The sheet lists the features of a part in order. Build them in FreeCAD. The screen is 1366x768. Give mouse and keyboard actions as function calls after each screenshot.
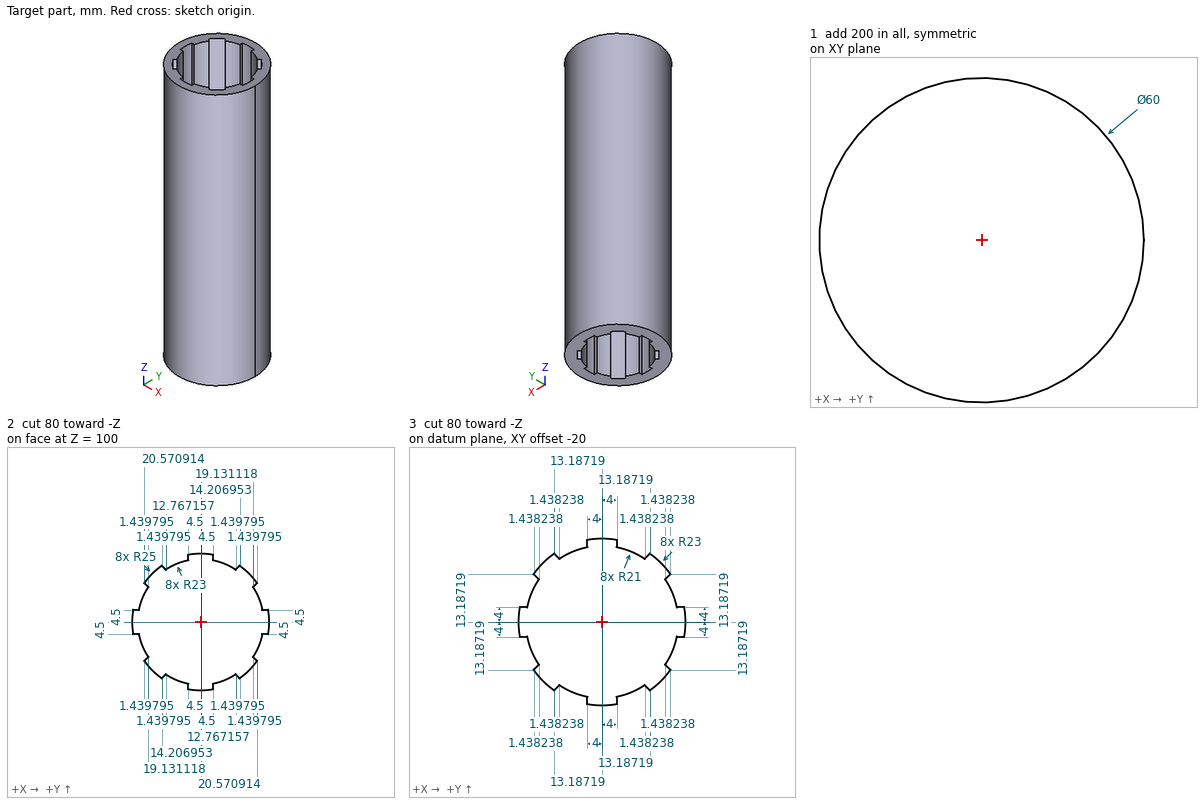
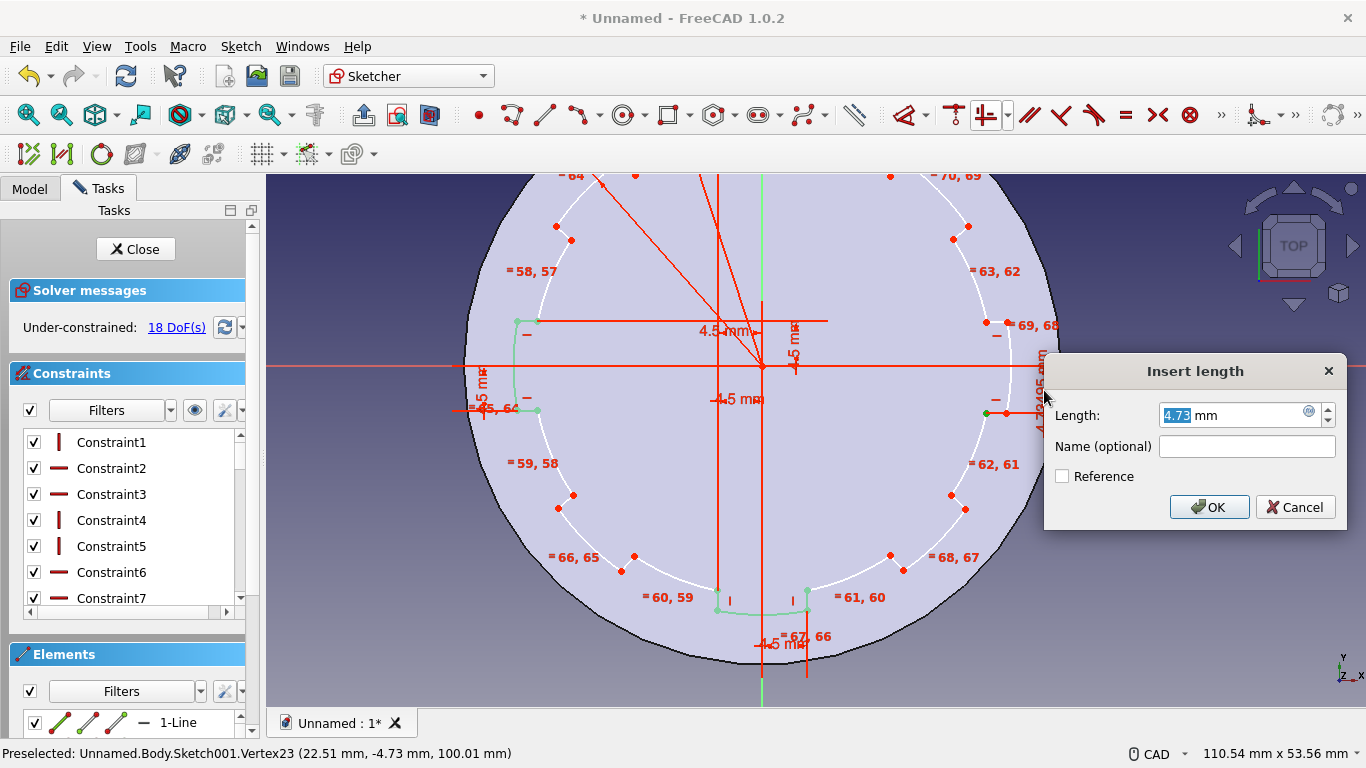
text(4.5)
key(Return)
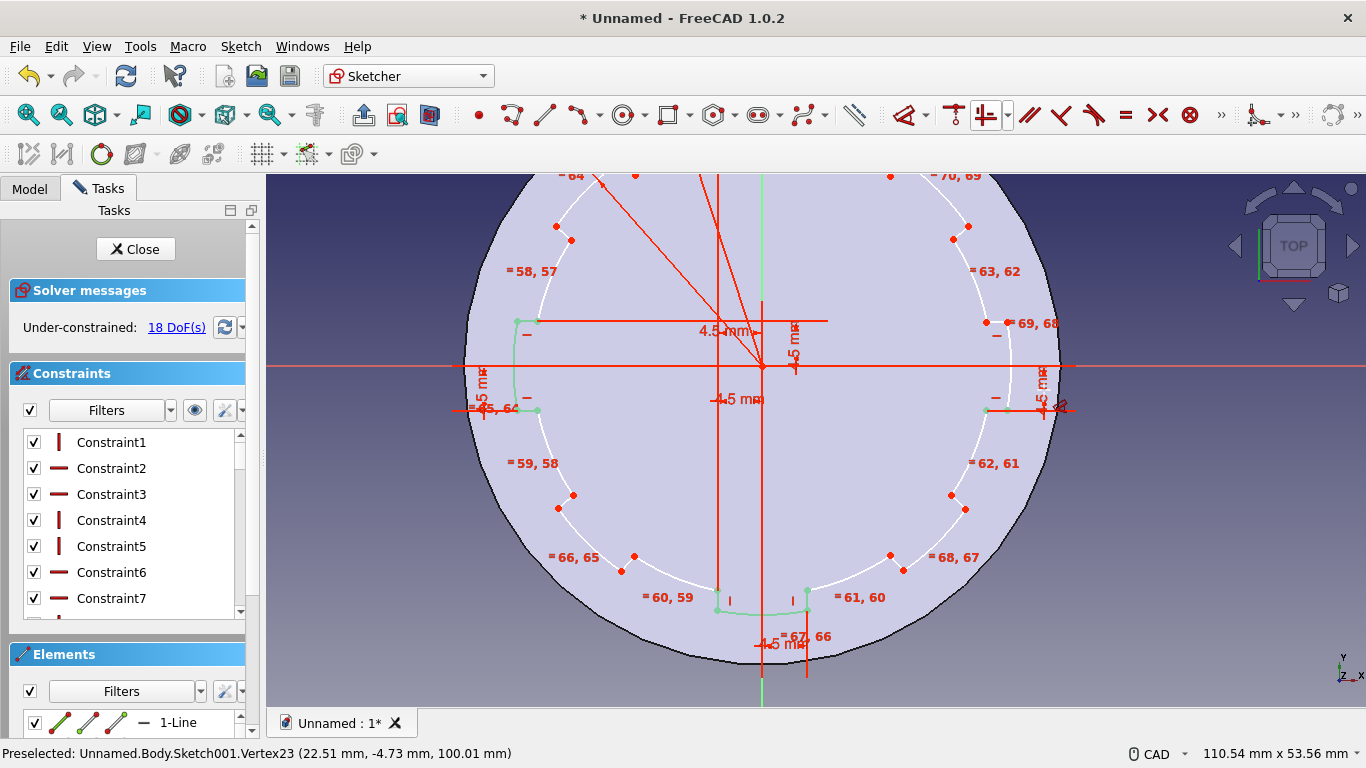
click(1007, 322)
click(1041, 344)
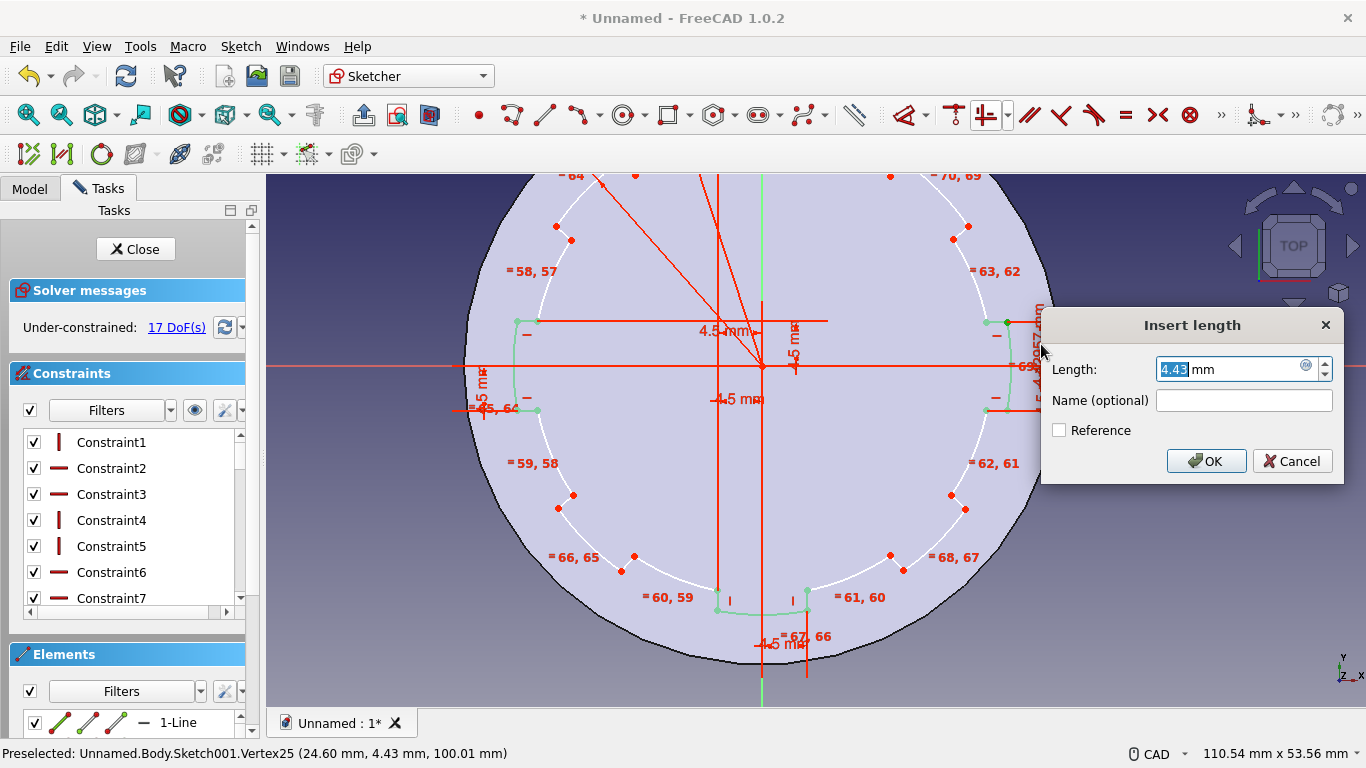
text(4.5)
key(Return)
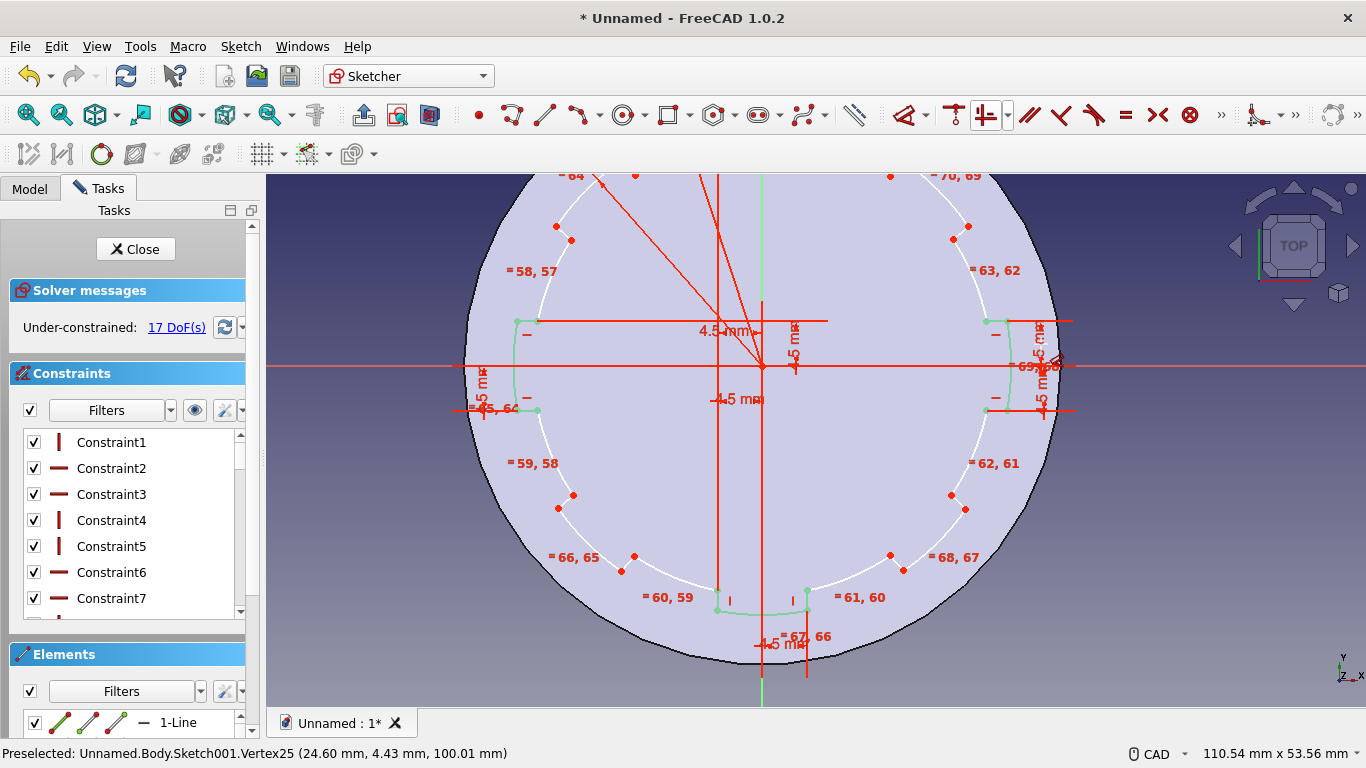
scroll(717, 592, down, 2)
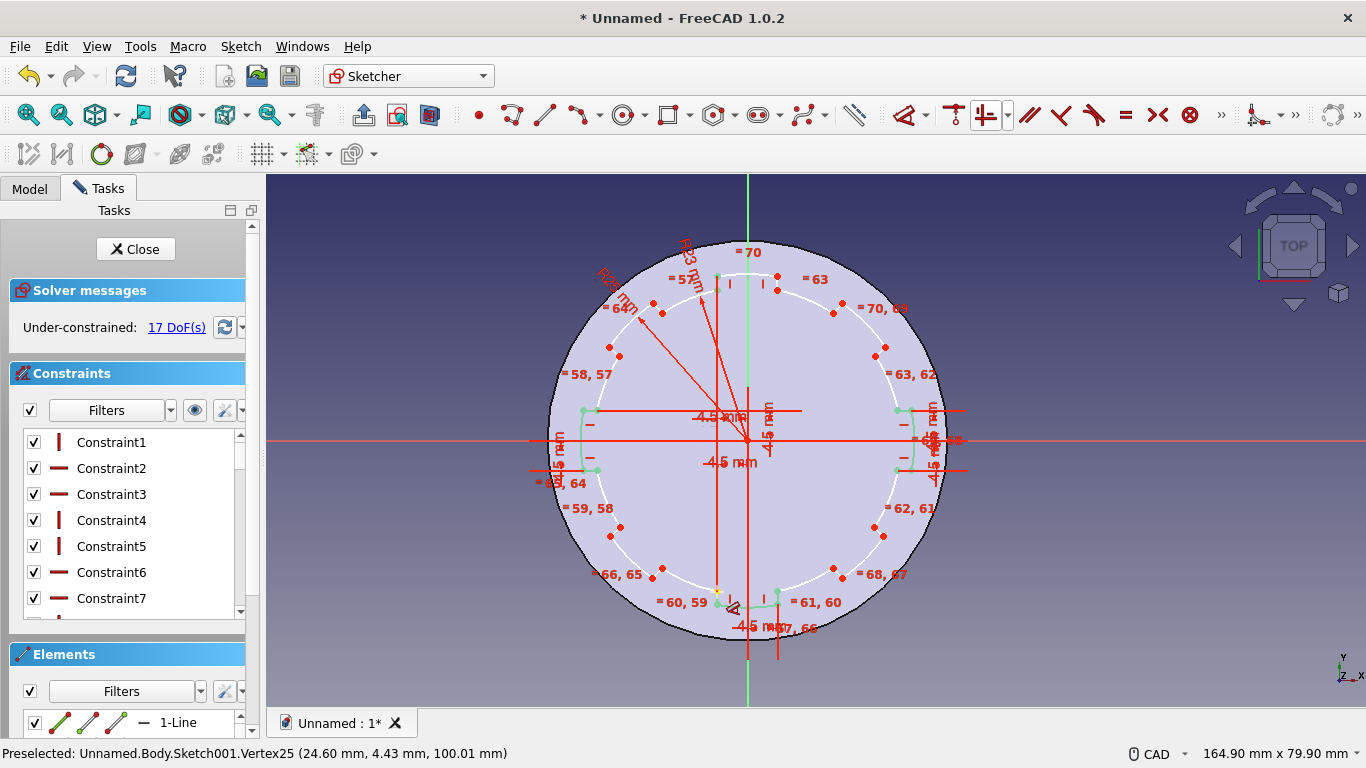
scroll(777, 290, up, 2)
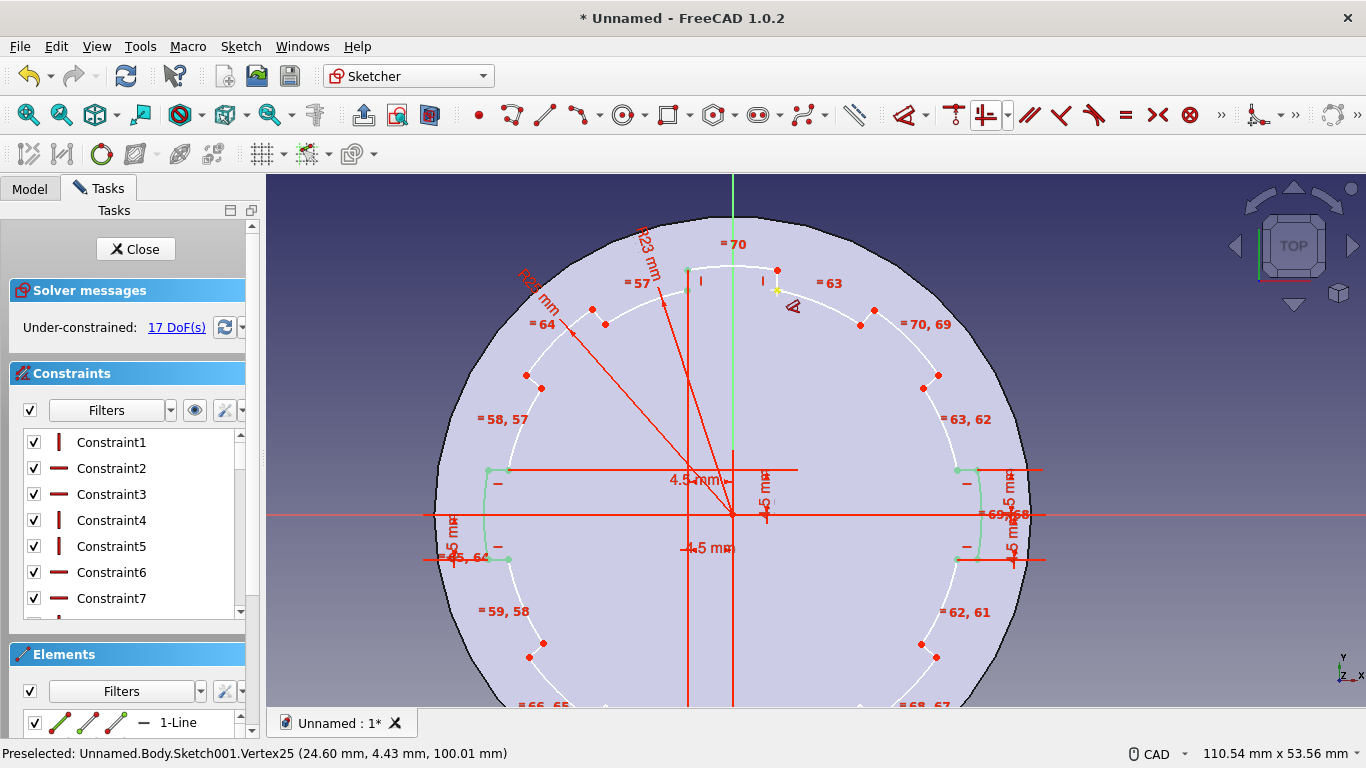
click(777, 290)
click(755, 232)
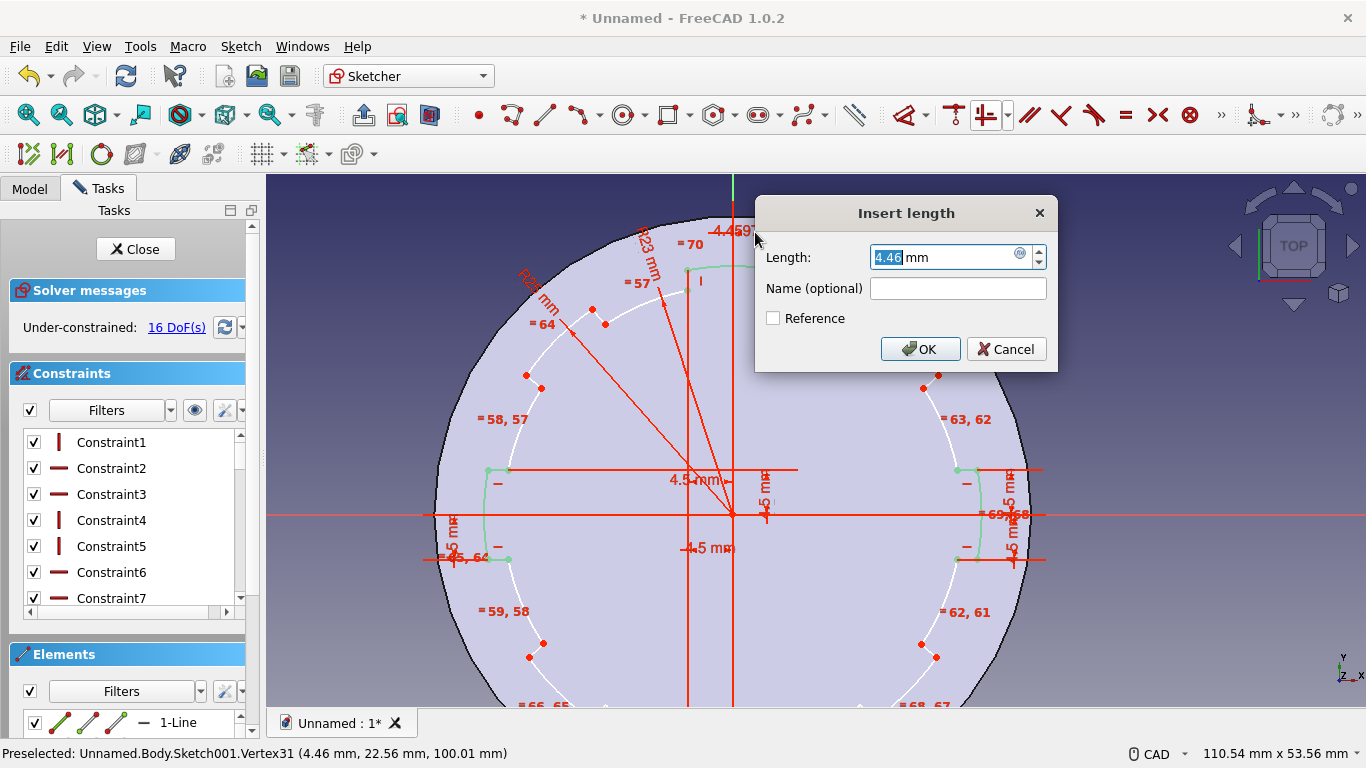
text(4.5)
key(Return)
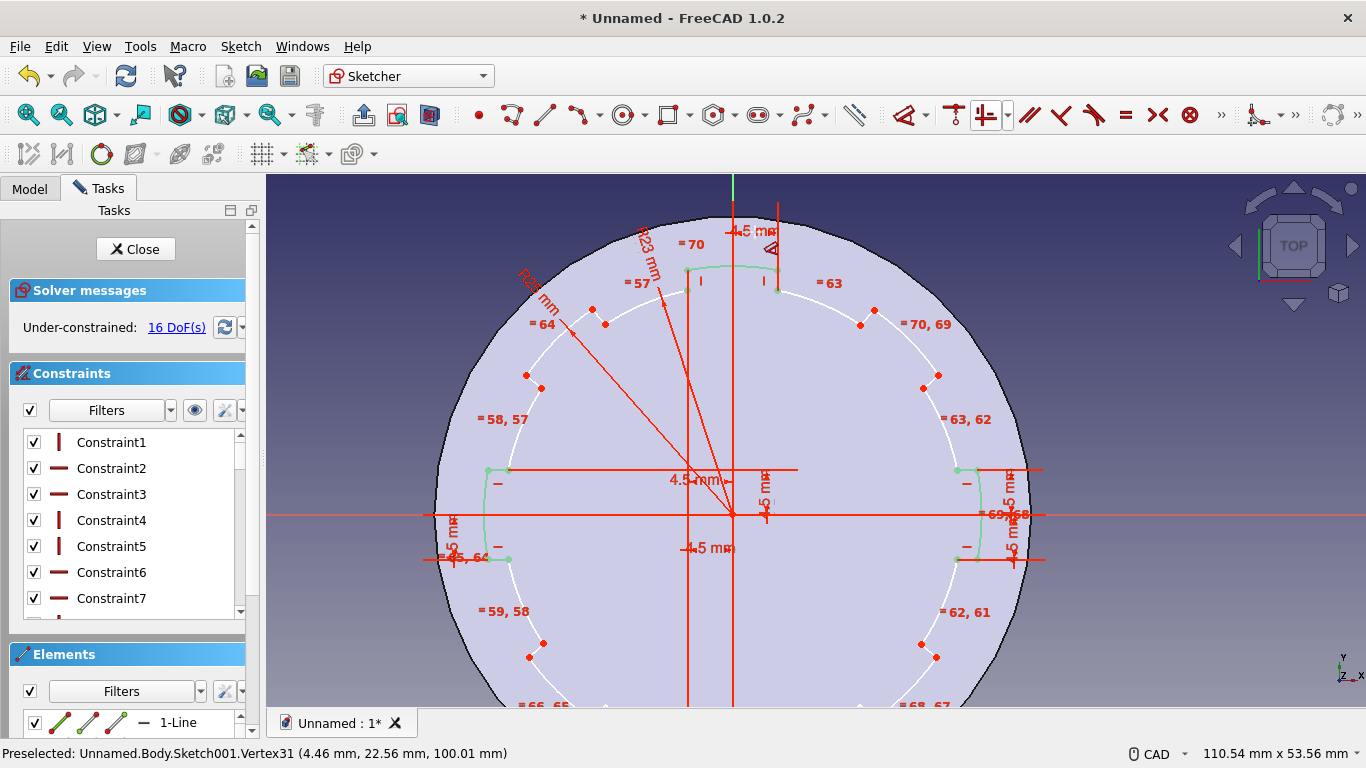
scroll(599, 317, up, 6)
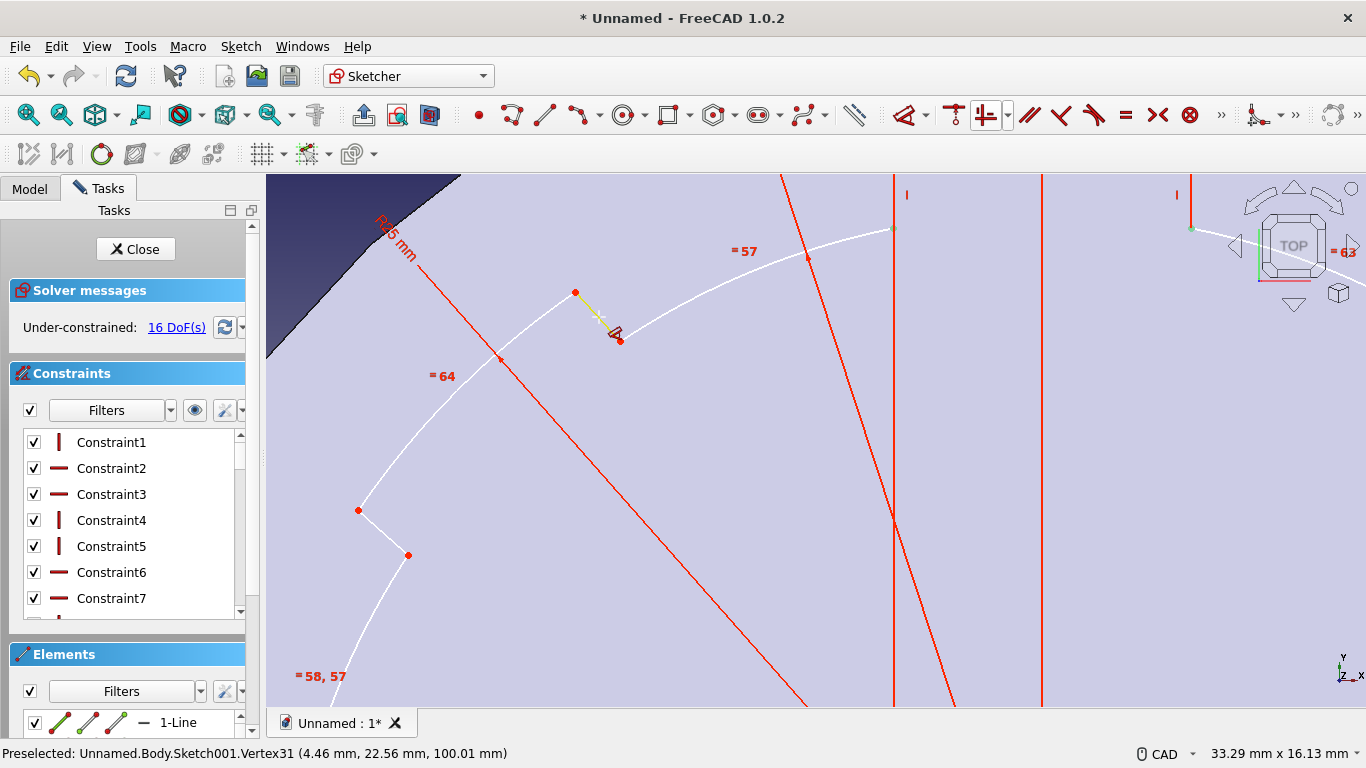
click(598, 317)
click(598, 258)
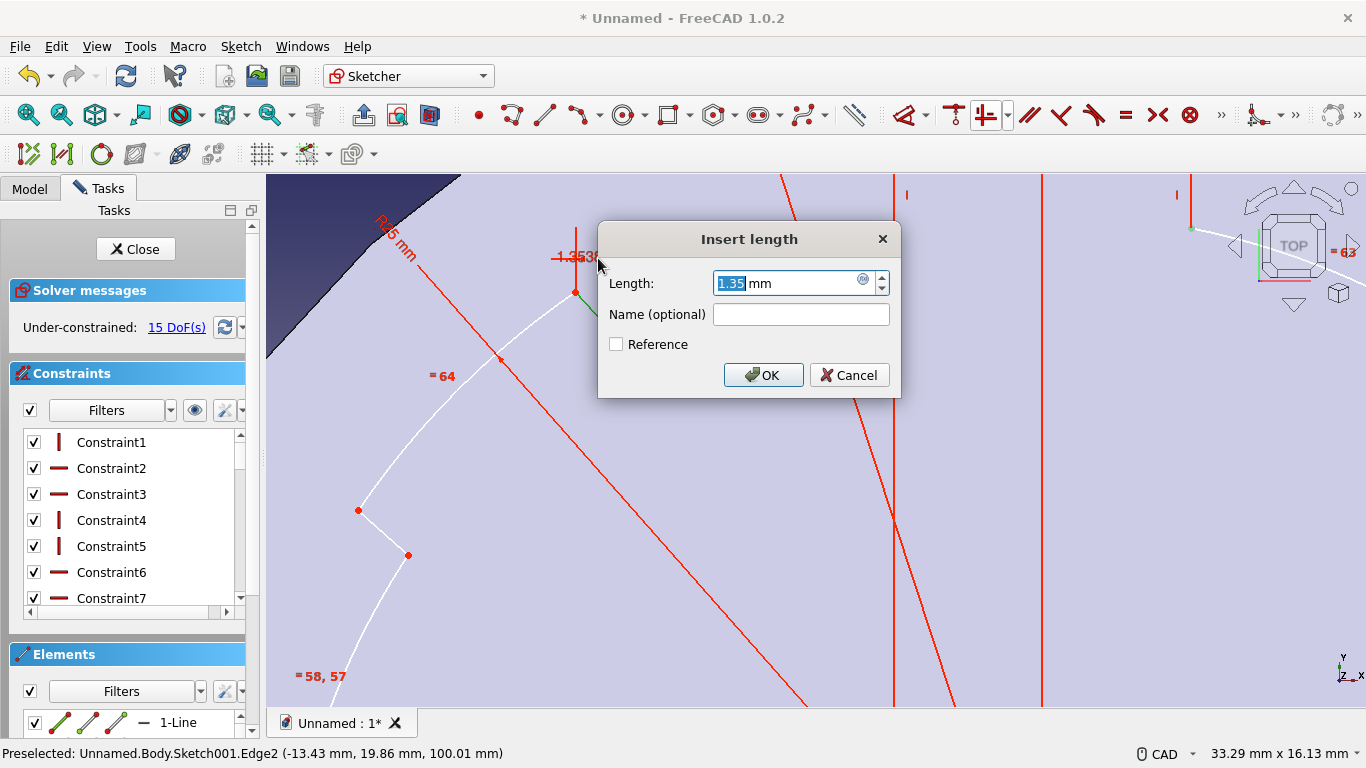
text(1.439795)
key(Return)